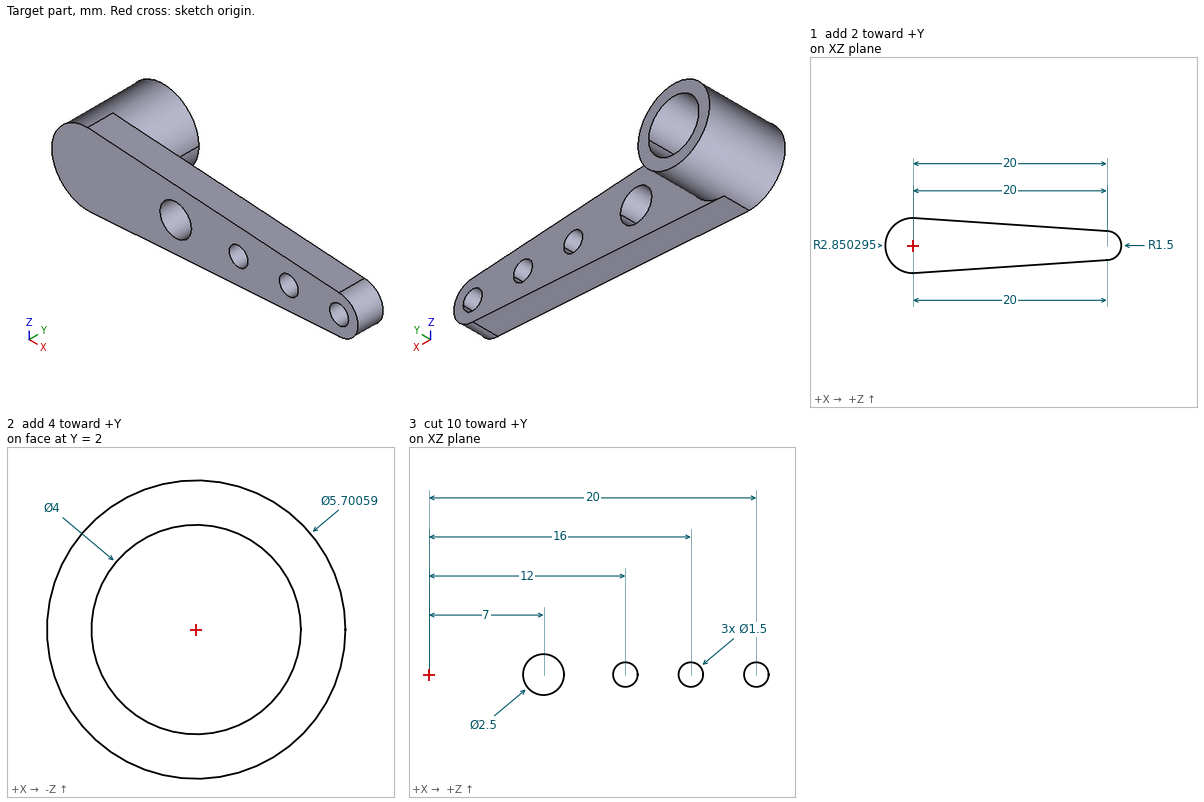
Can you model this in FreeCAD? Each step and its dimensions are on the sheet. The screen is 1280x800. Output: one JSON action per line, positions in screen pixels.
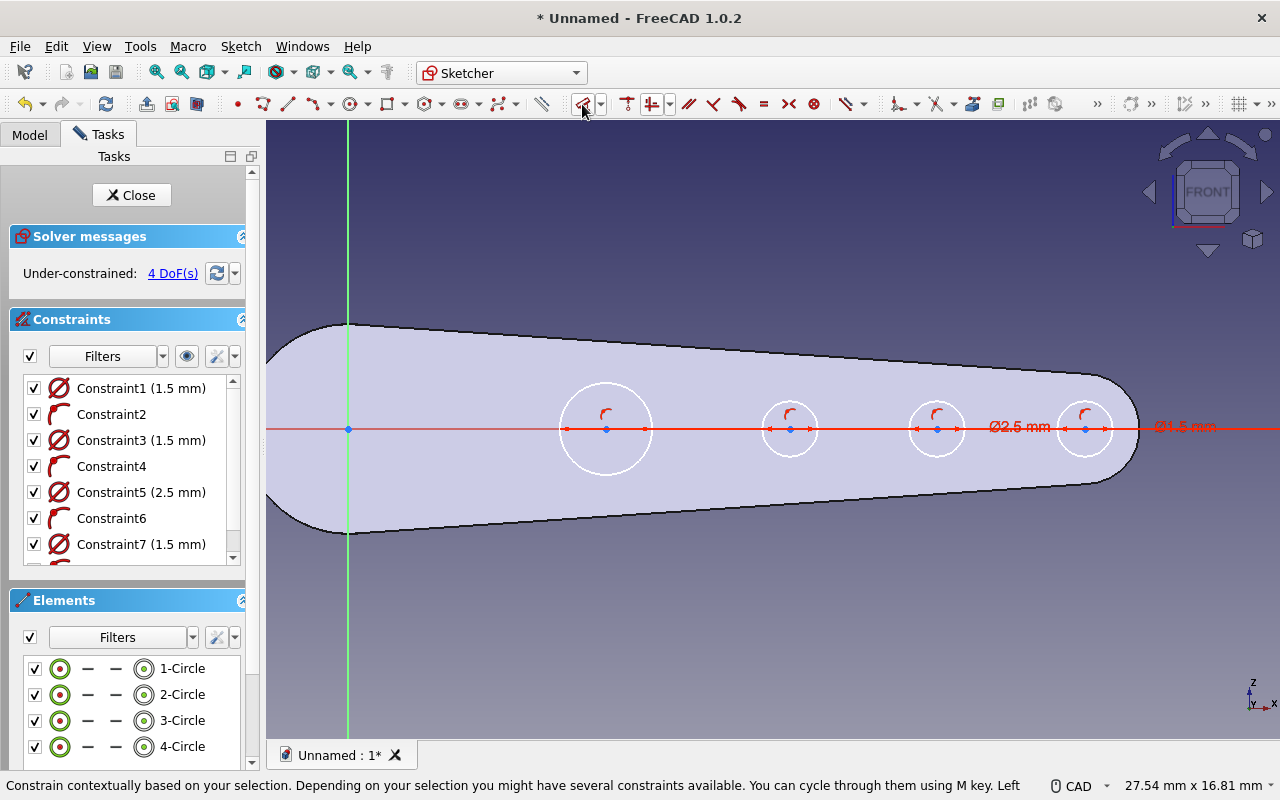
{"action": "left_click", "coordinate": [606, 429]}
{"action": "left_click", "coordinate": [477, 463]}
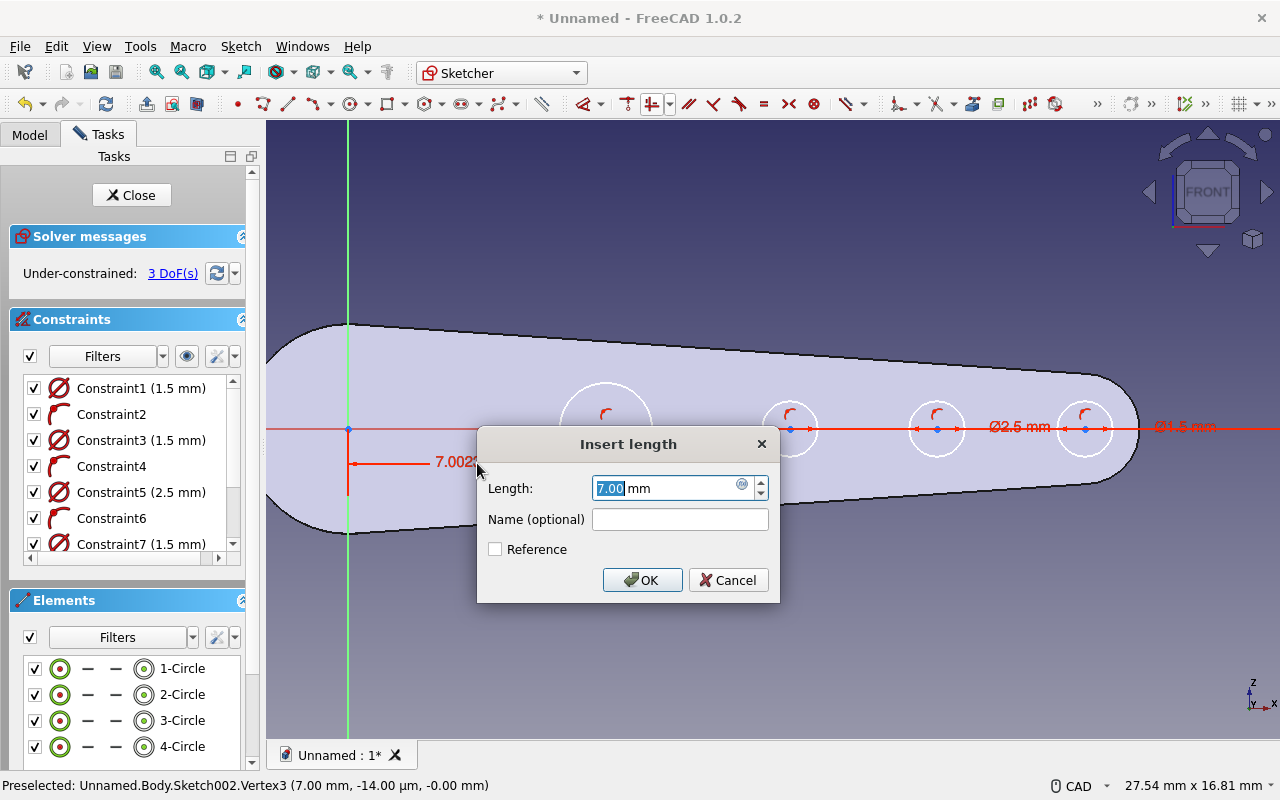
{"action": "type", "text": "7"}
{"action": "key", "text": "Return"}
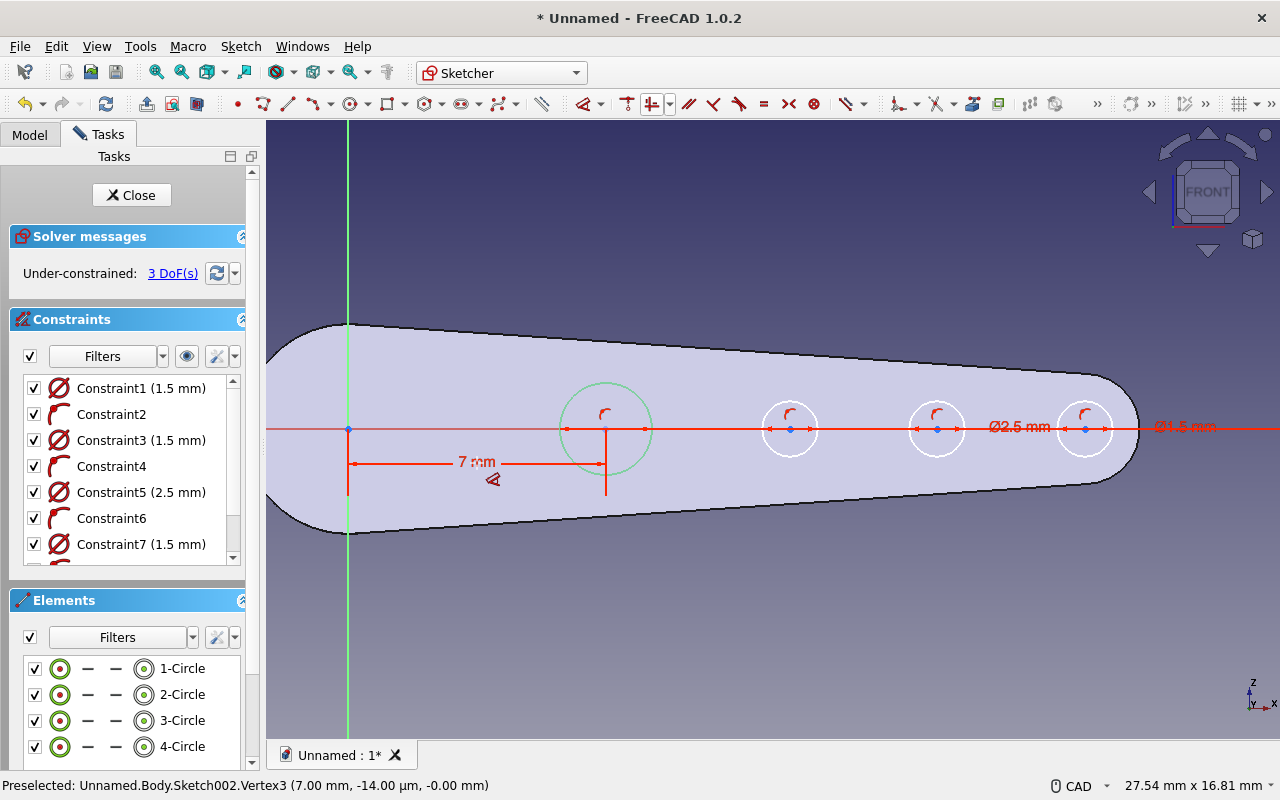
{"action": "left_click", "coordinate": [937, 429]}
{"action": "left_click", "coordinate": [849, 463]}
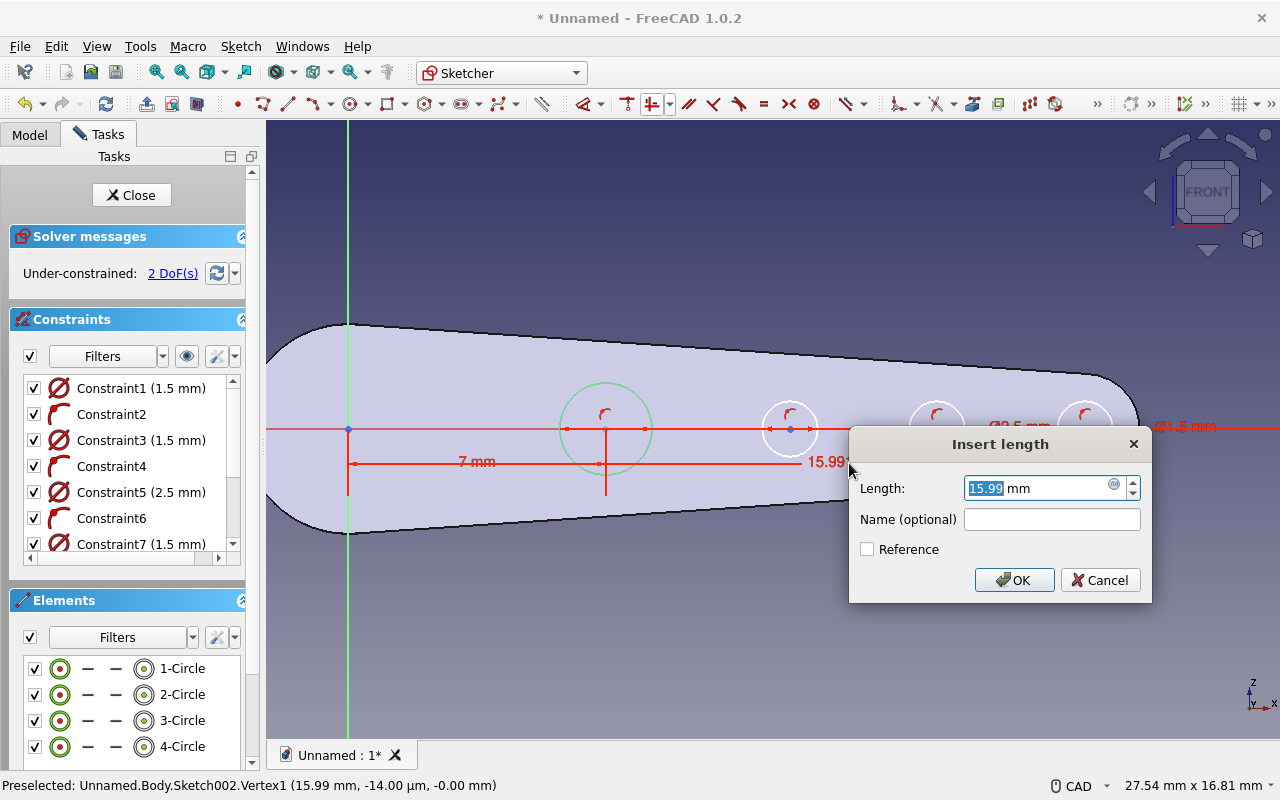
{"action": "type", "text": "16"}
{"action": "key", "text": "Return"}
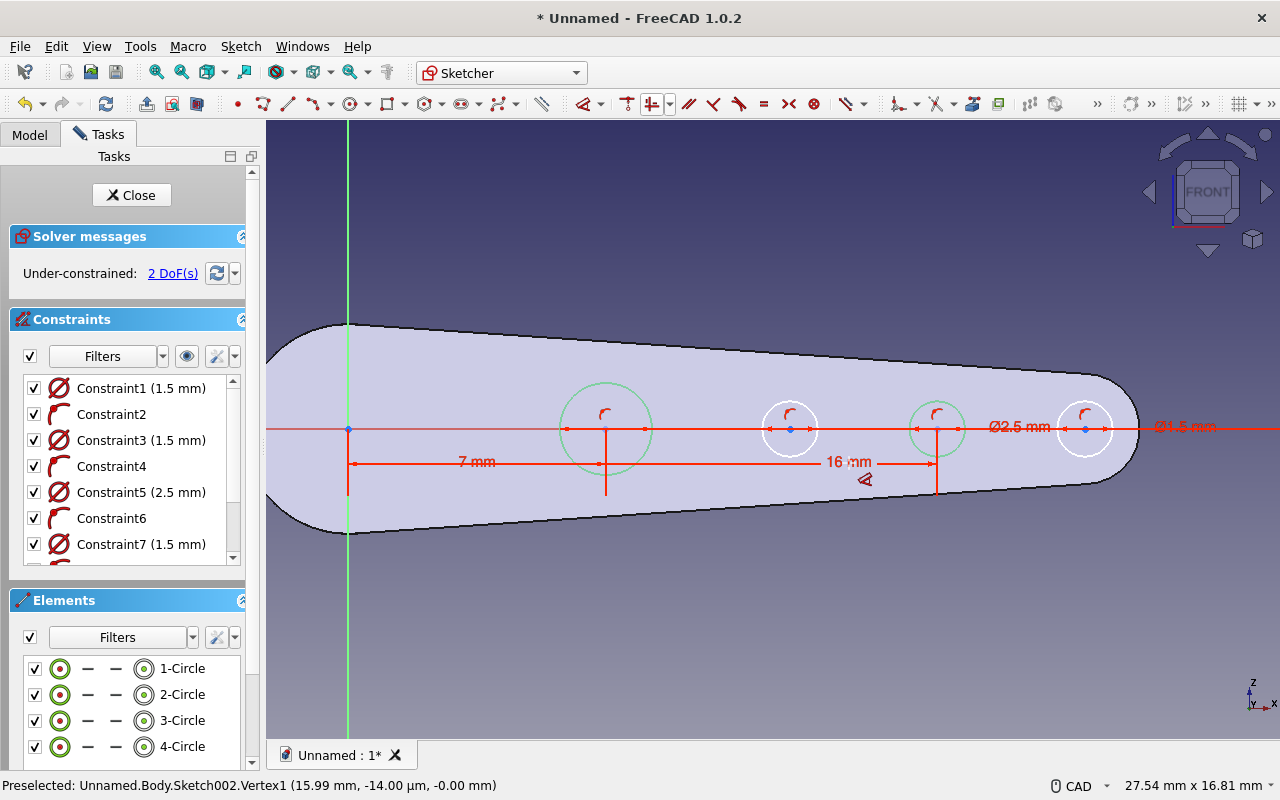
{"action": "left_click", "coordinate": [790, 429]}
{"action": "left_click", "coordinate": [671, 463]}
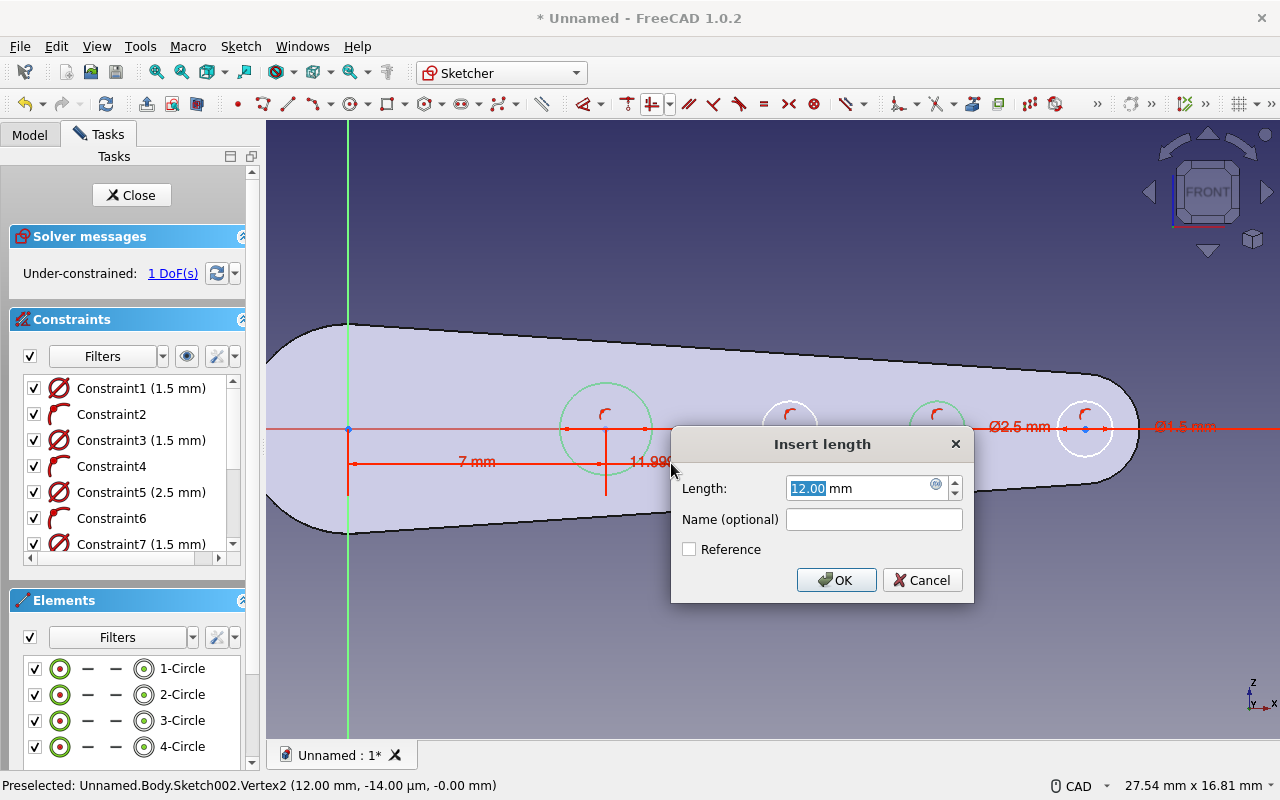
{"action": "type", "text": "12"}
{"action": "key", "text": "Return"}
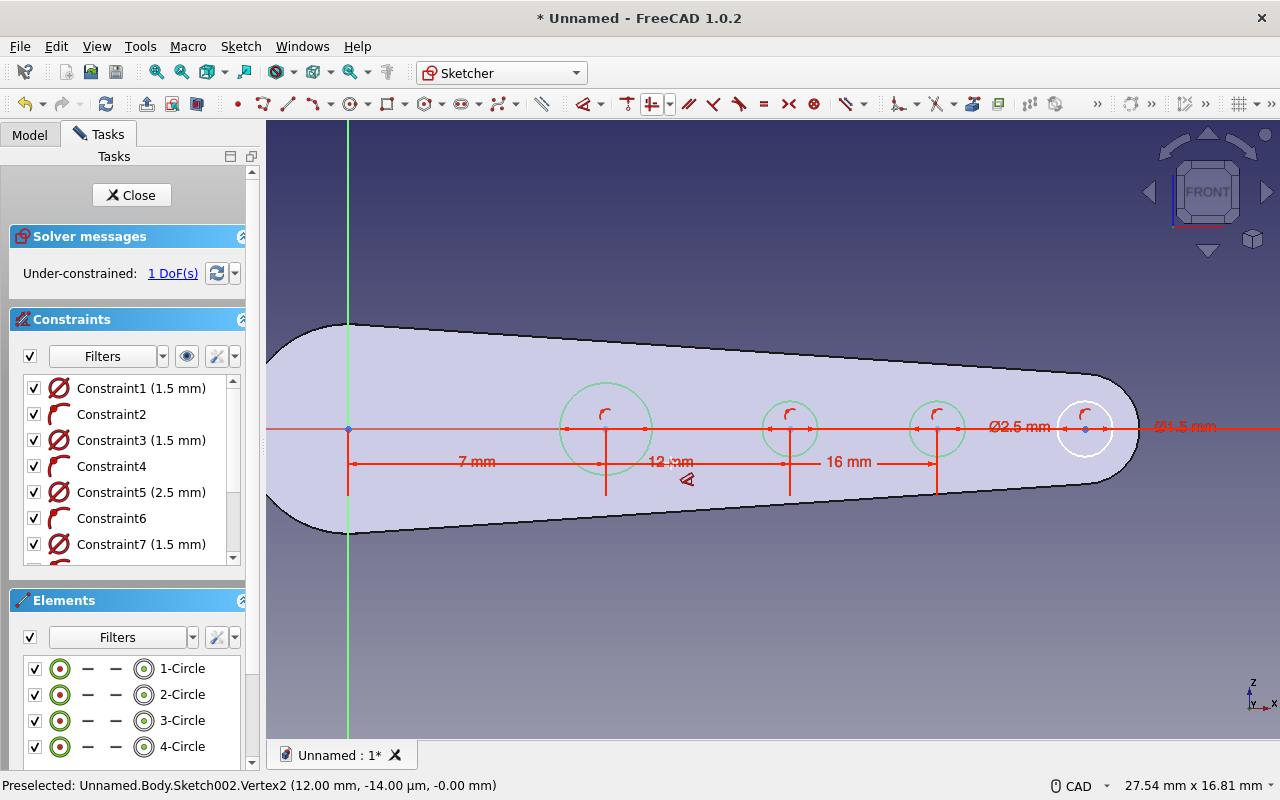
{"action": "left_click", "coordinate": [1085, 429]}
{"action": "left_click", "coordinate": [547, 463]}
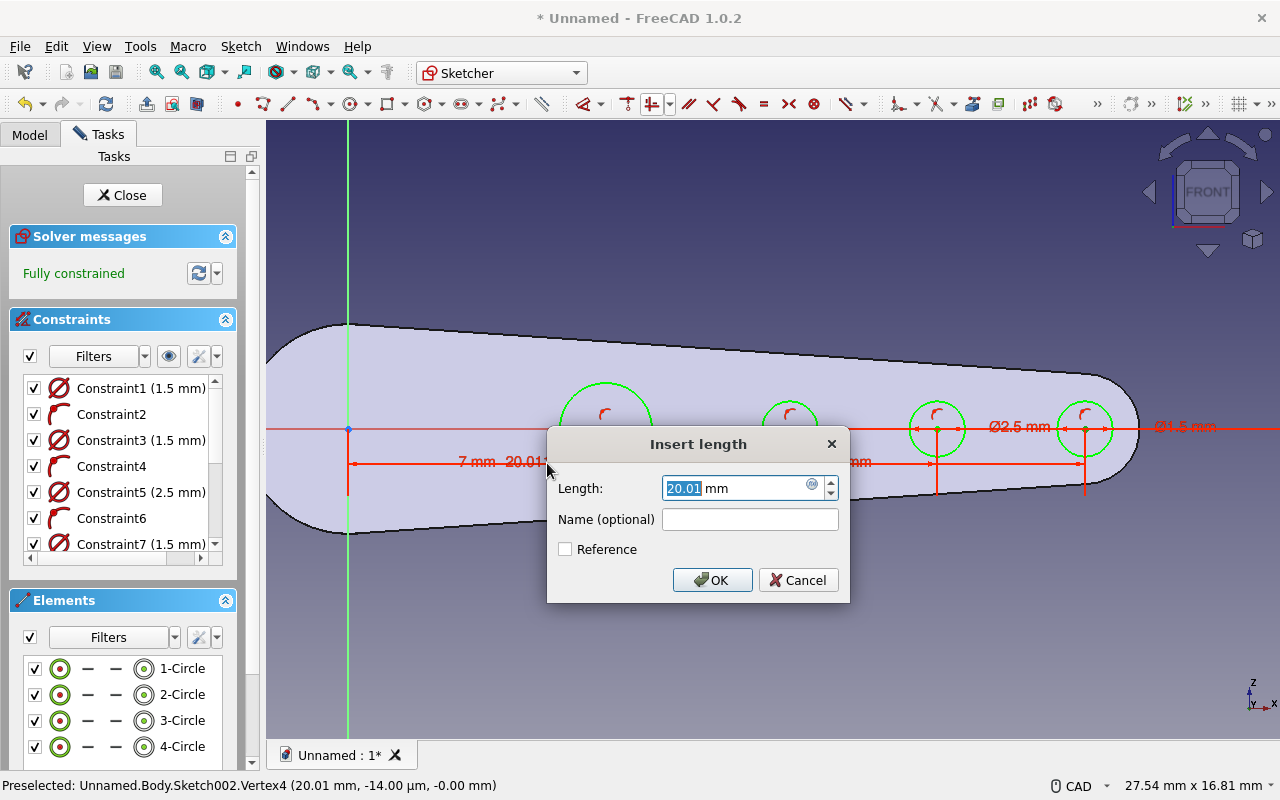
{"action": "type", "text": "20"}
{"action": "key", "text": "Return"}
{"action": "key", "text": "Escape"}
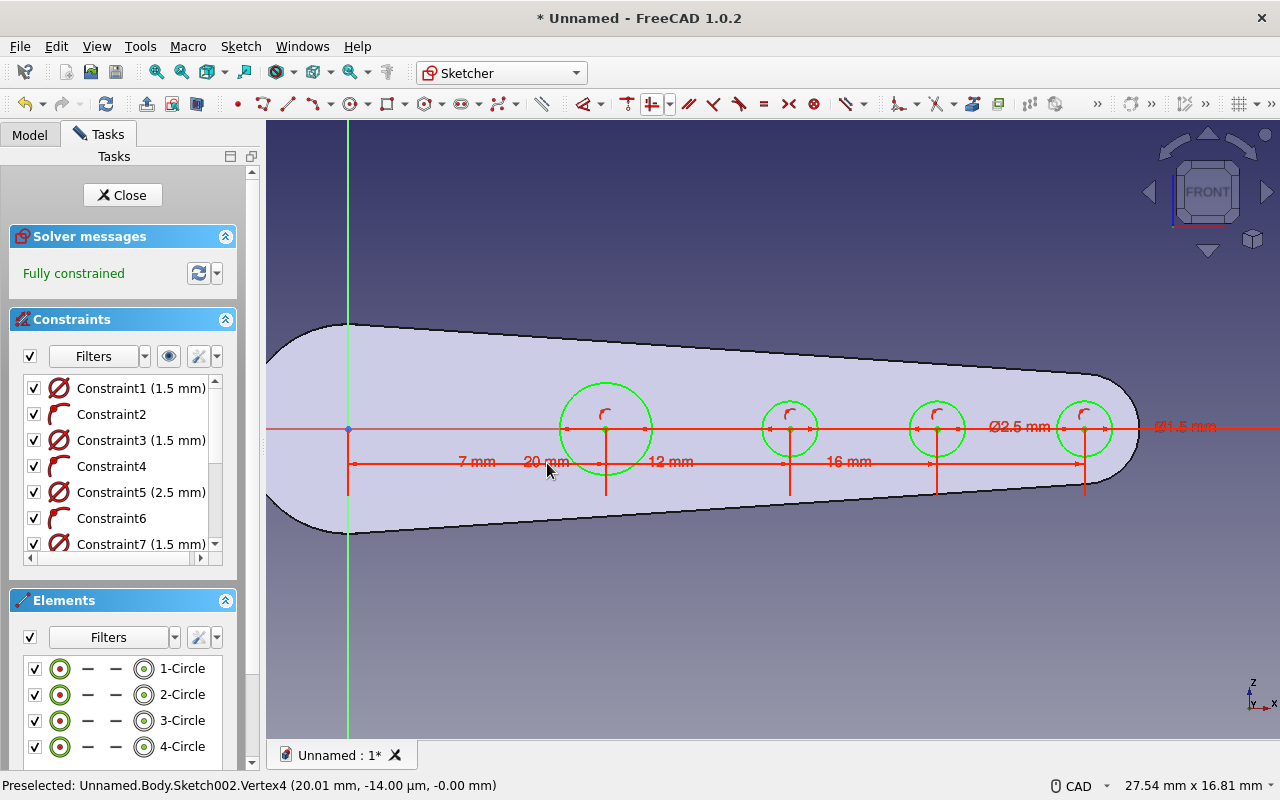
{"action": "left_click", "coordinate": [123, 195]}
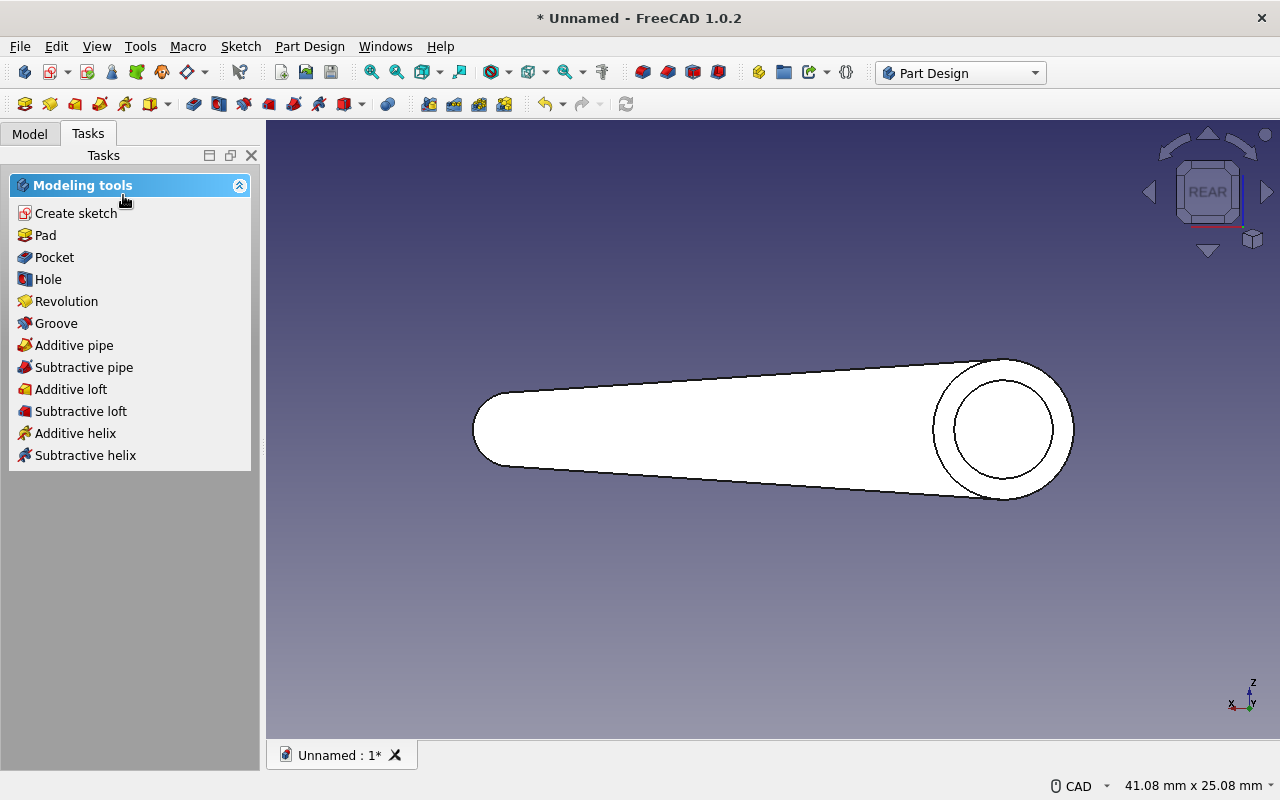
{"action": "left_click", "coordinate": [194, 104]}